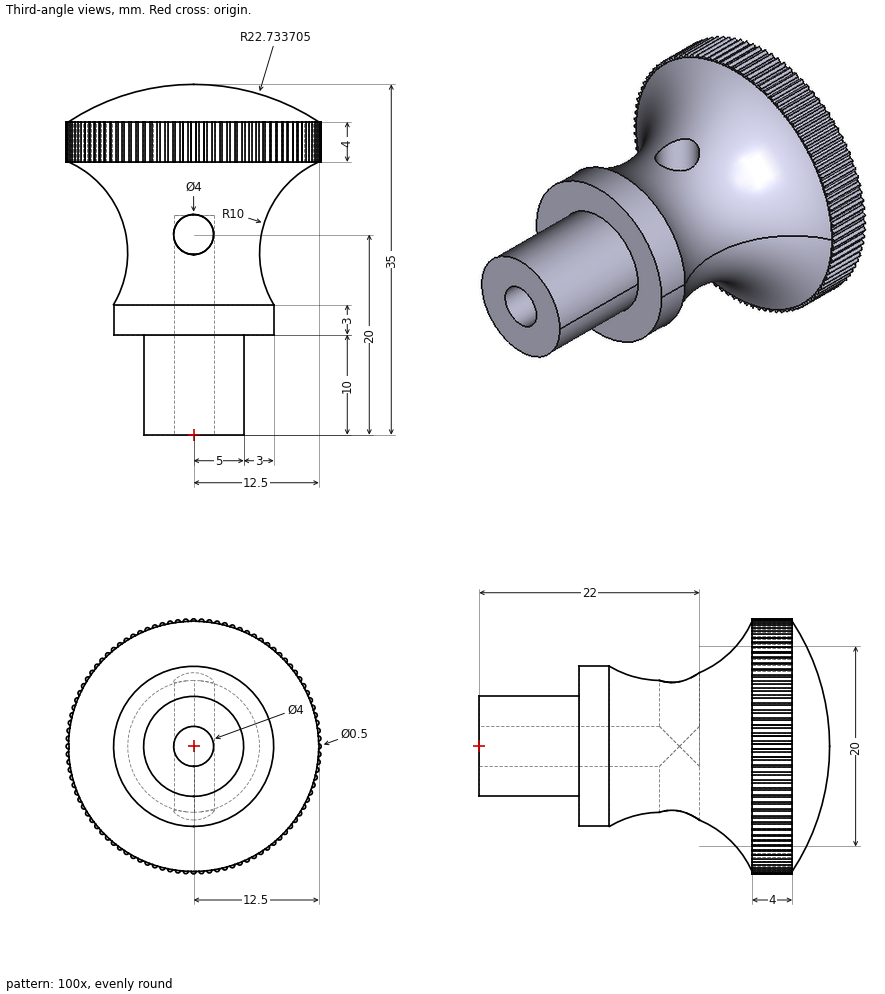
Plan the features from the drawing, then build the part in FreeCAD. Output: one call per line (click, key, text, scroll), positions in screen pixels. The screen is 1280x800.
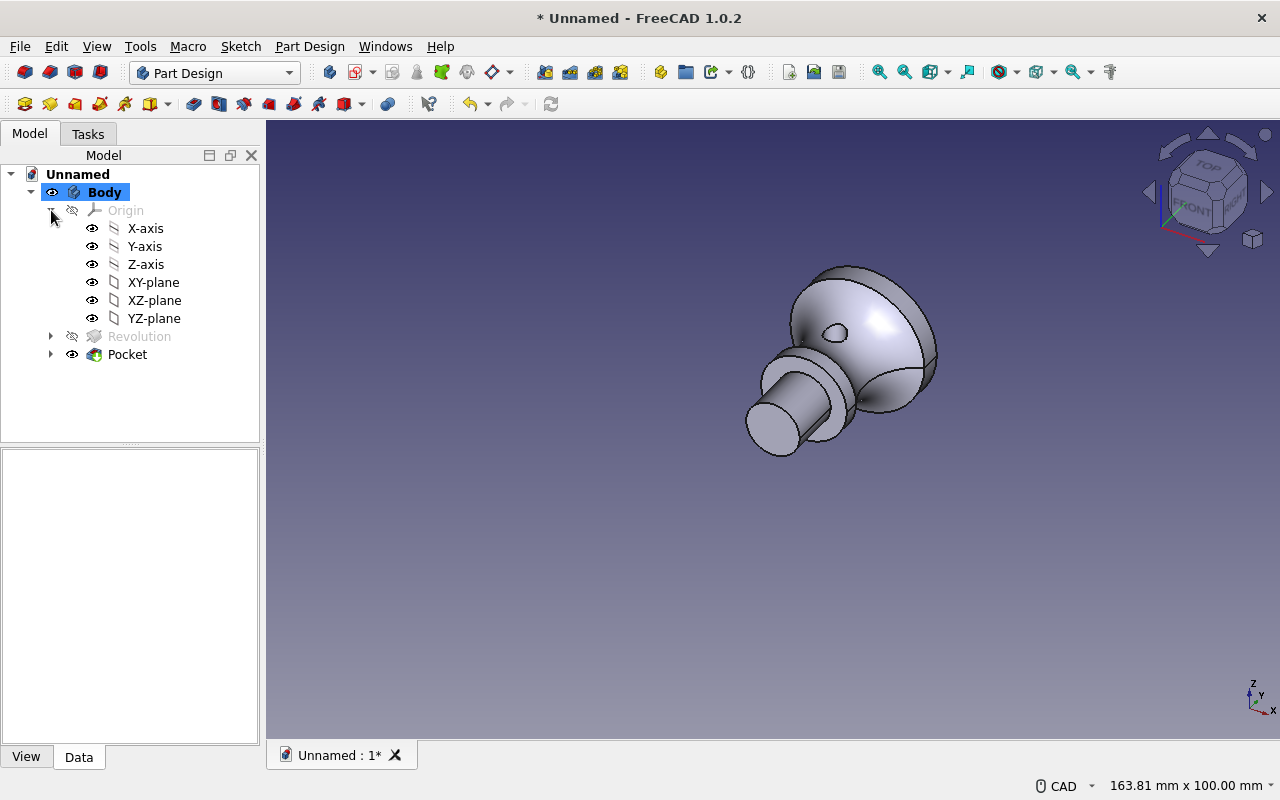
click(137, 300)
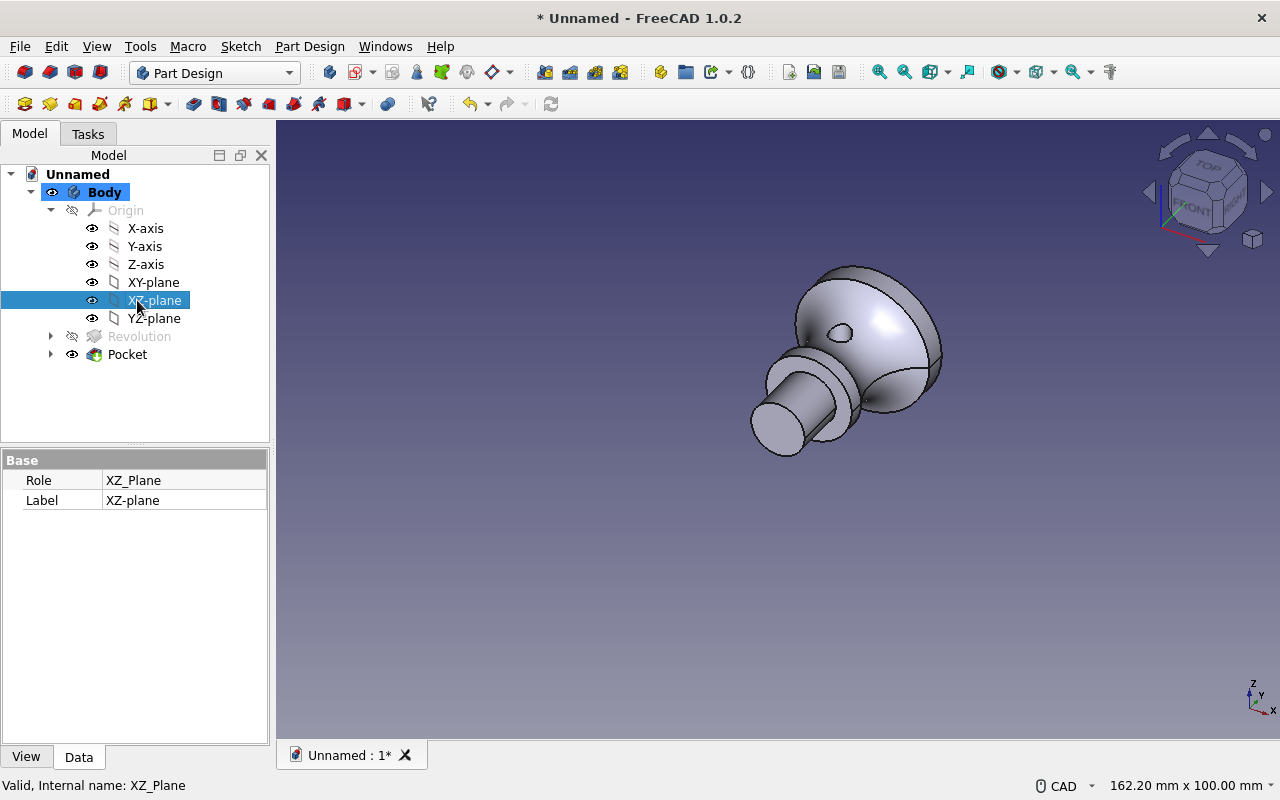
click(492, 72)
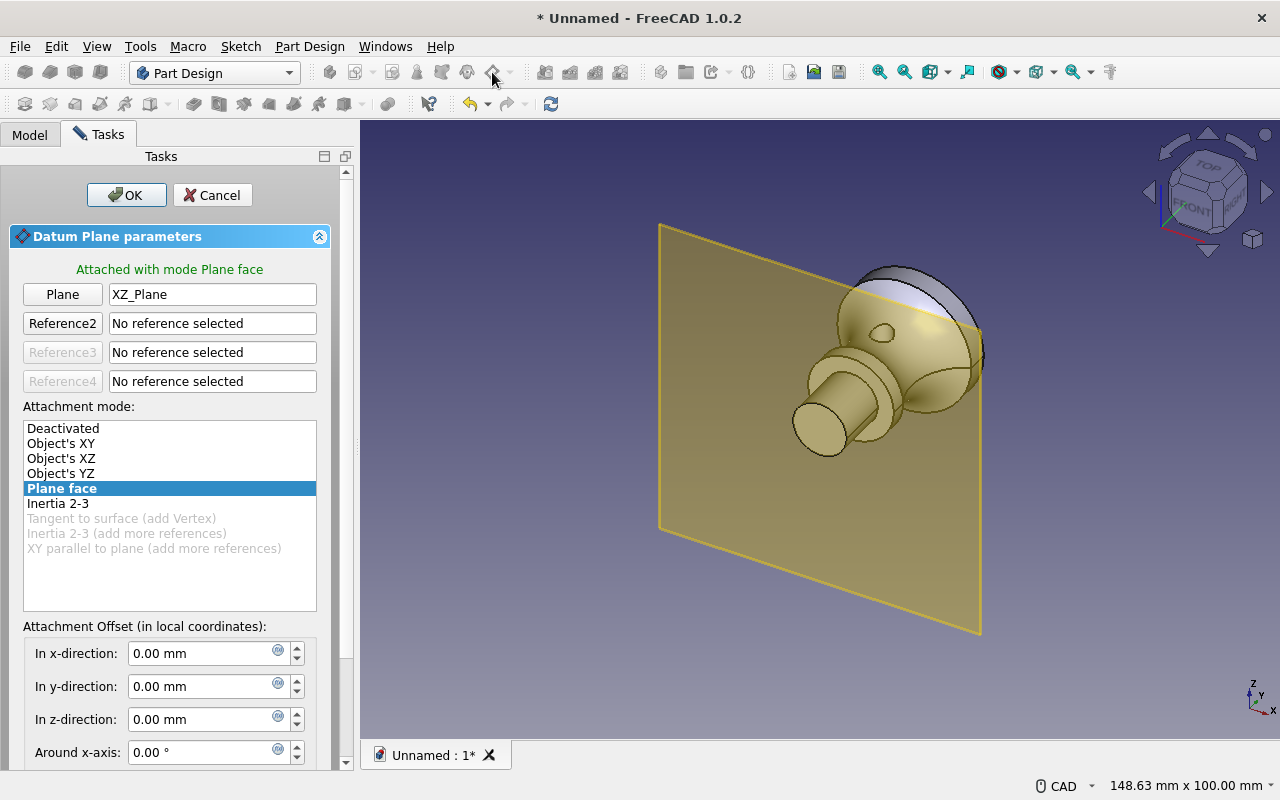
triple_click(210, 720)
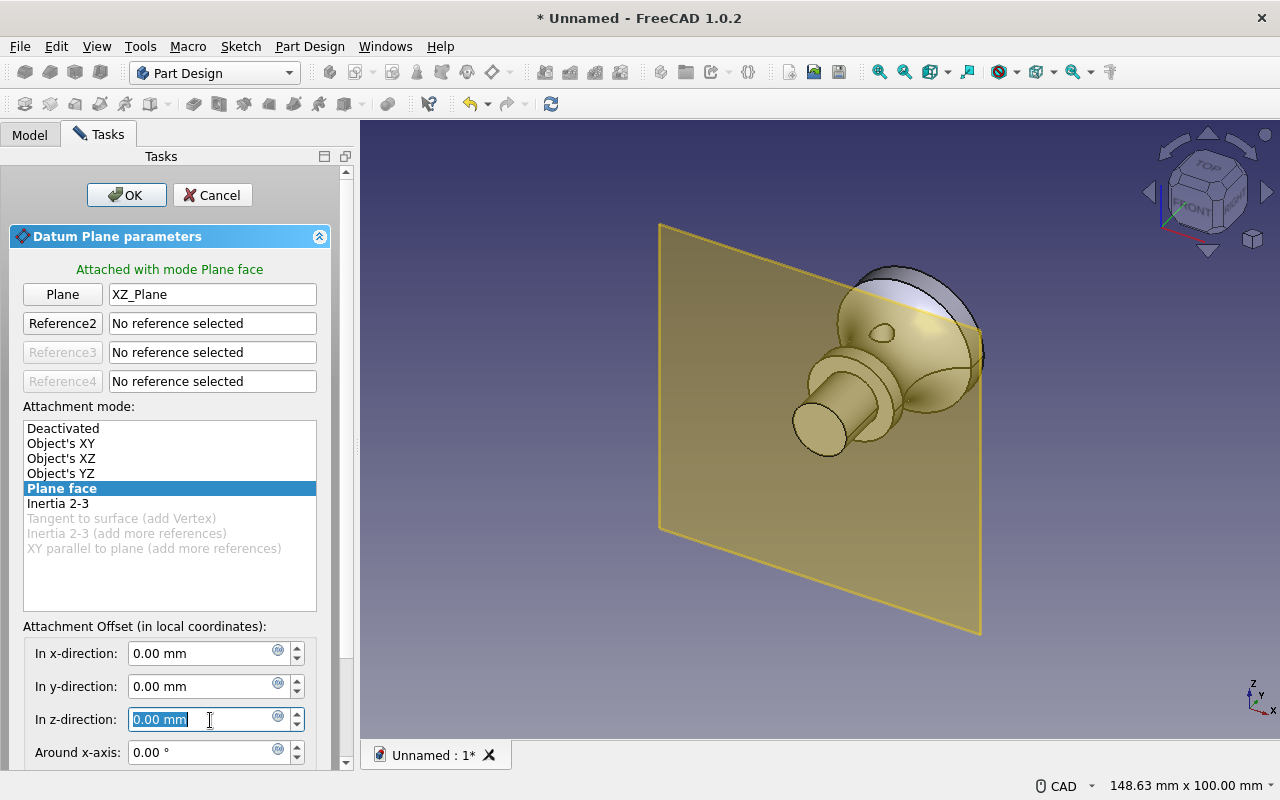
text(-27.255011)
key(Tab)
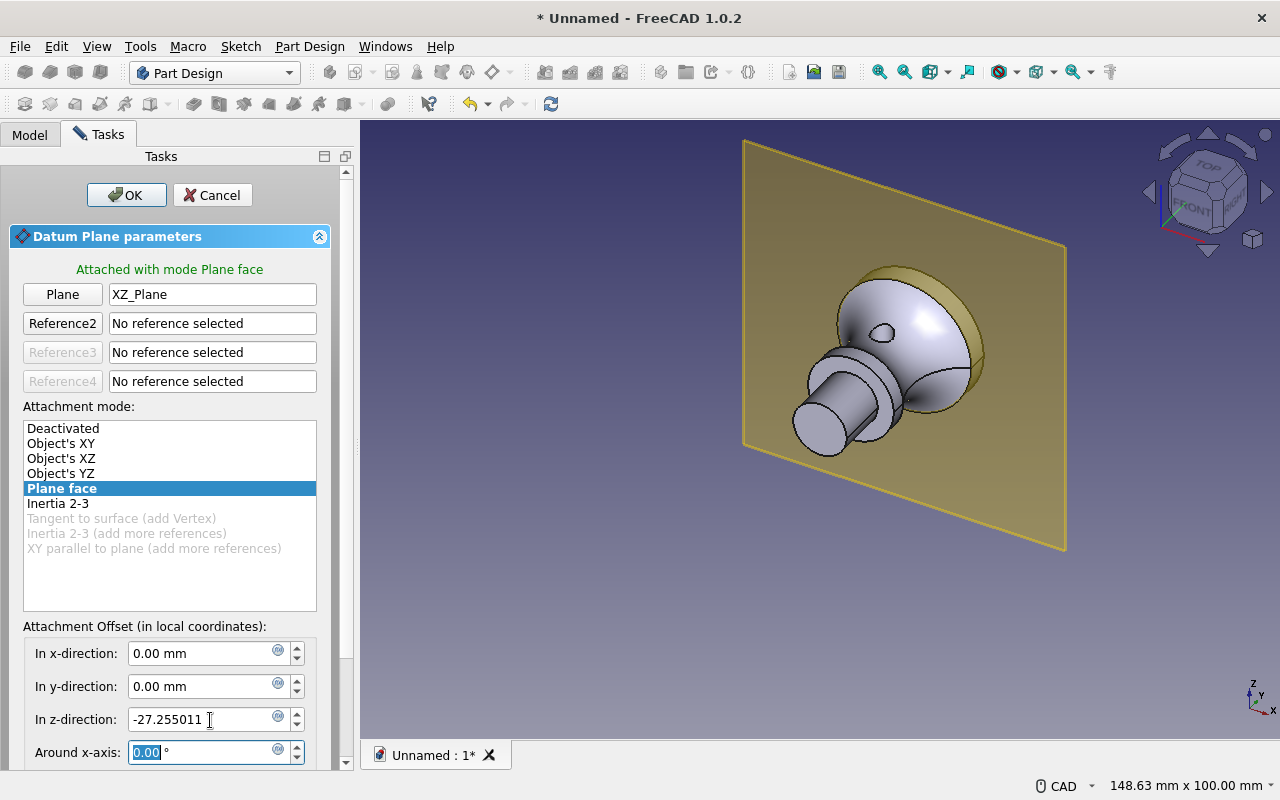
click(127, 195)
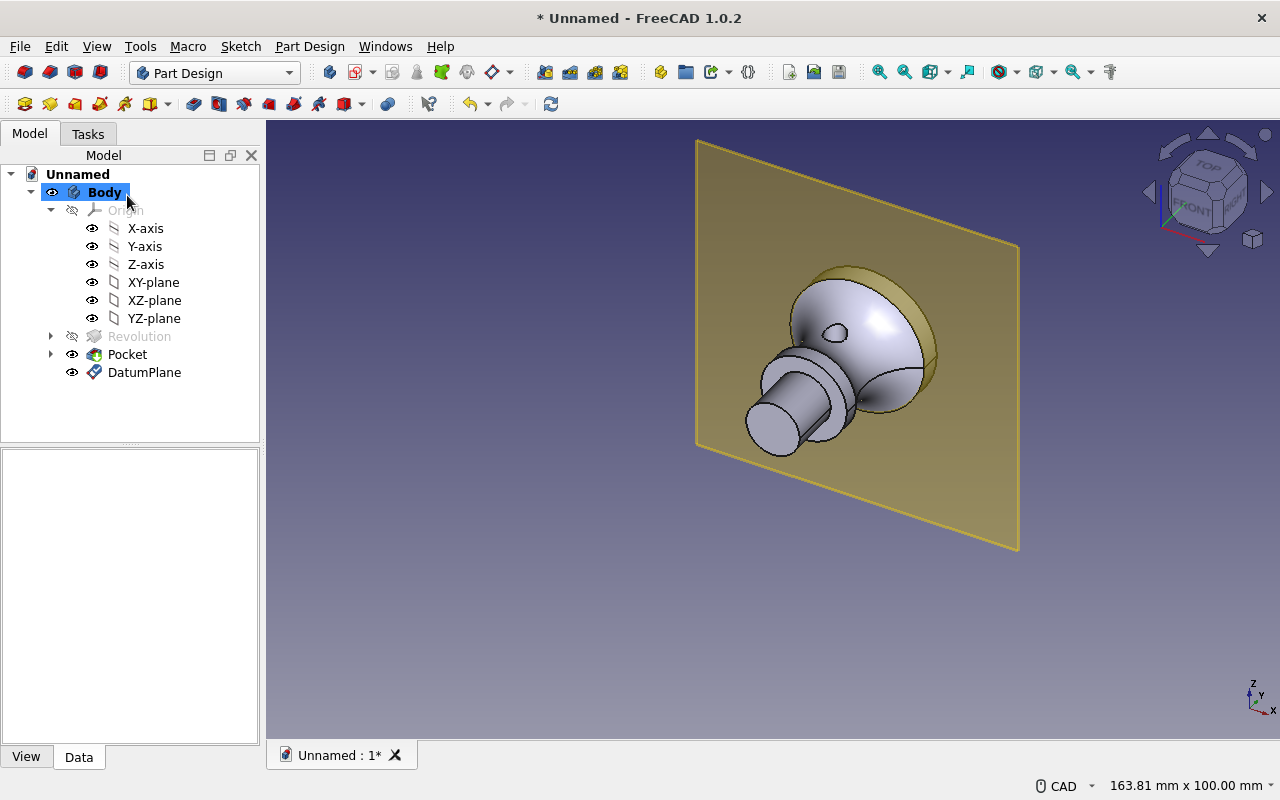
click(117, 372)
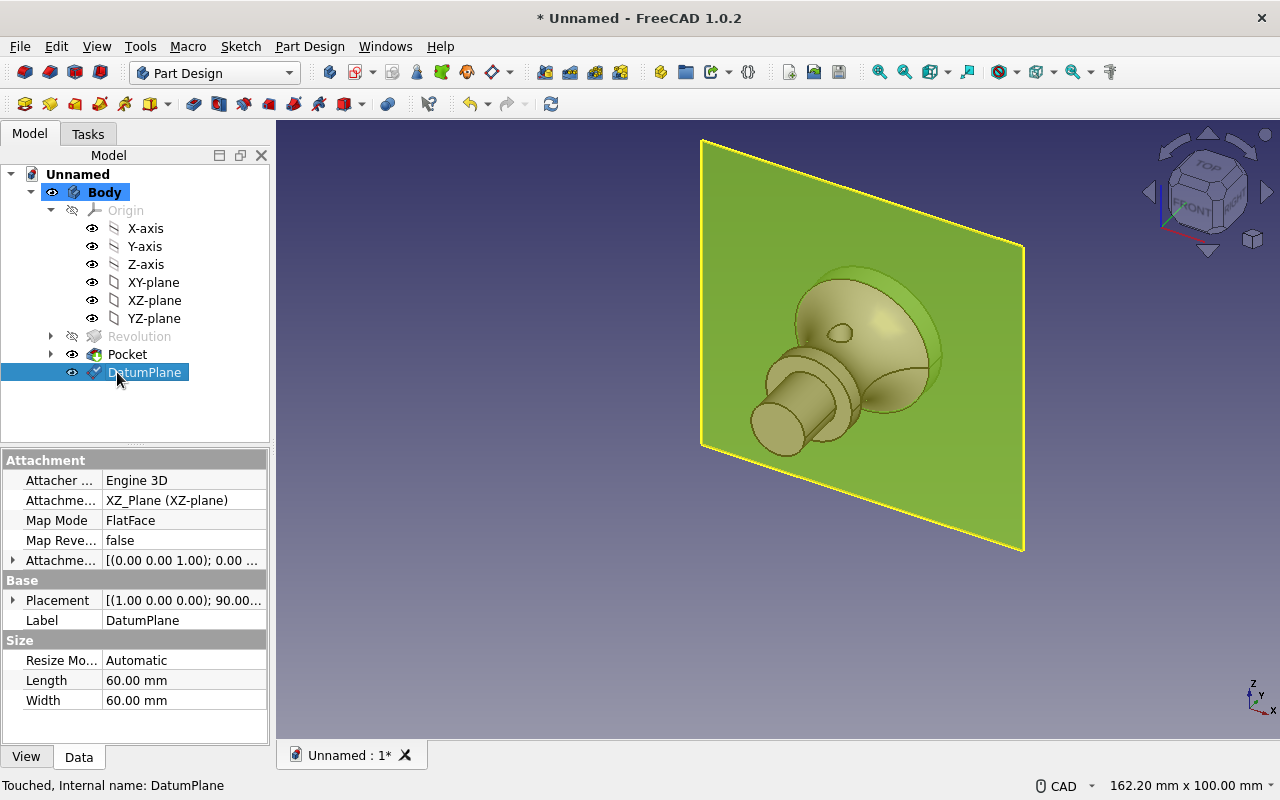
click(354, 72)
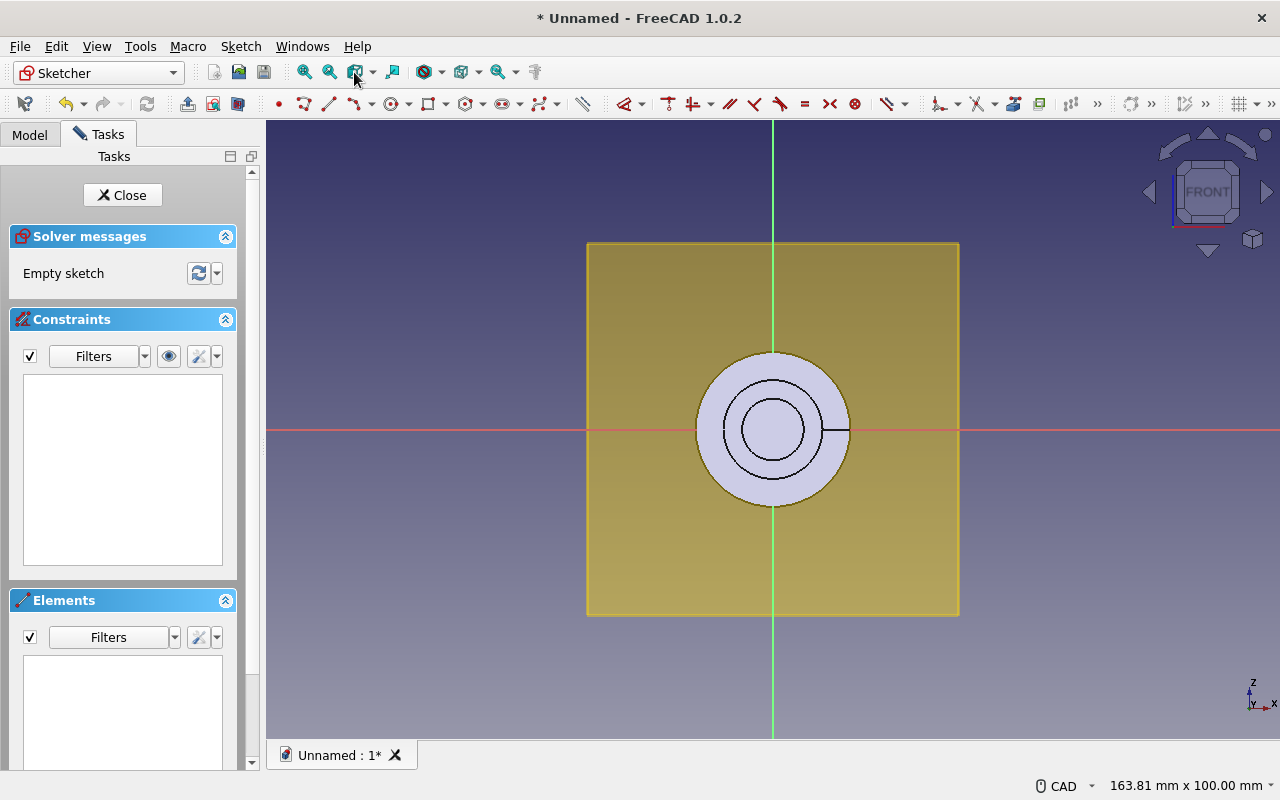
click(238, 104)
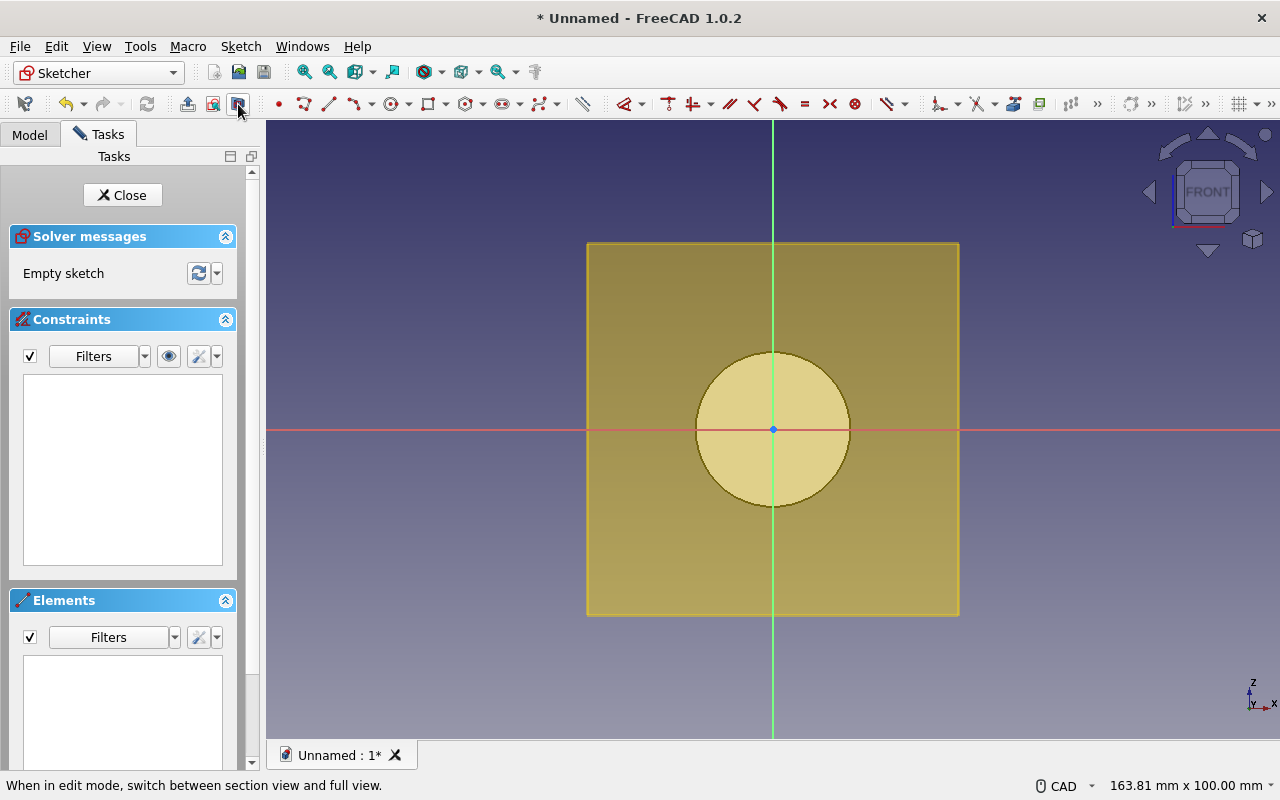
scroll(858, 430, up, 15)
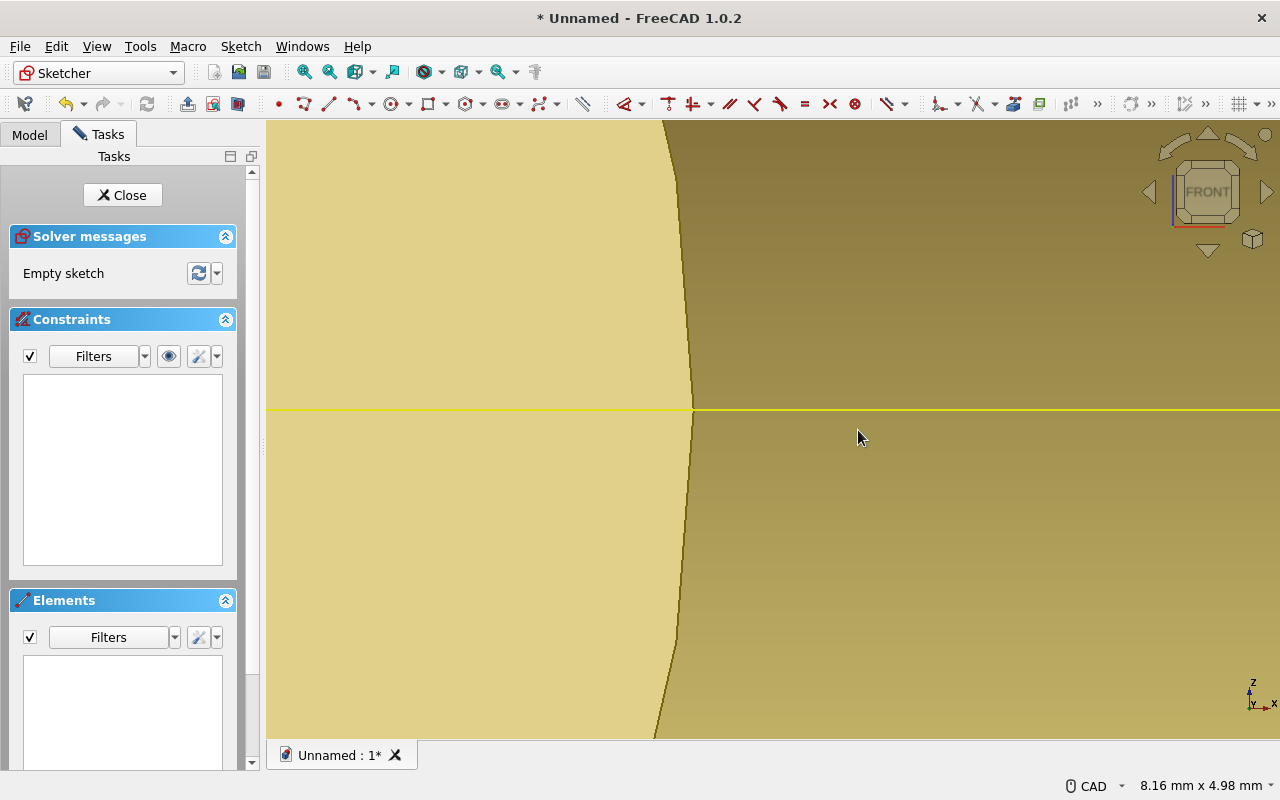
scroll(692, 407, up, 9)